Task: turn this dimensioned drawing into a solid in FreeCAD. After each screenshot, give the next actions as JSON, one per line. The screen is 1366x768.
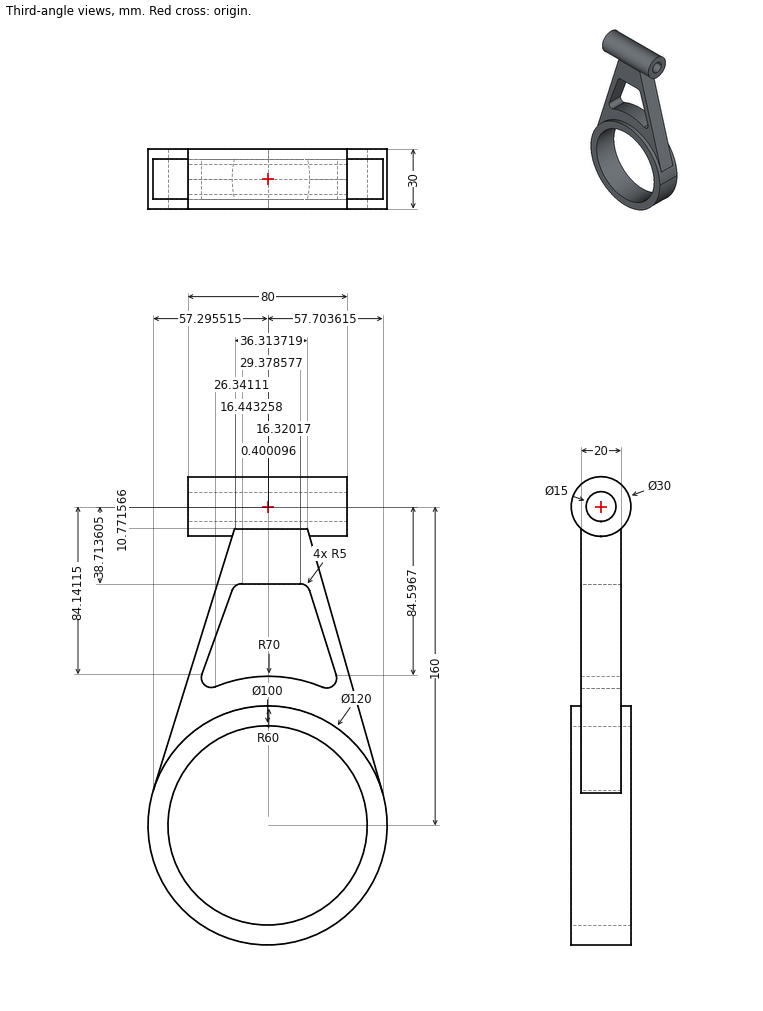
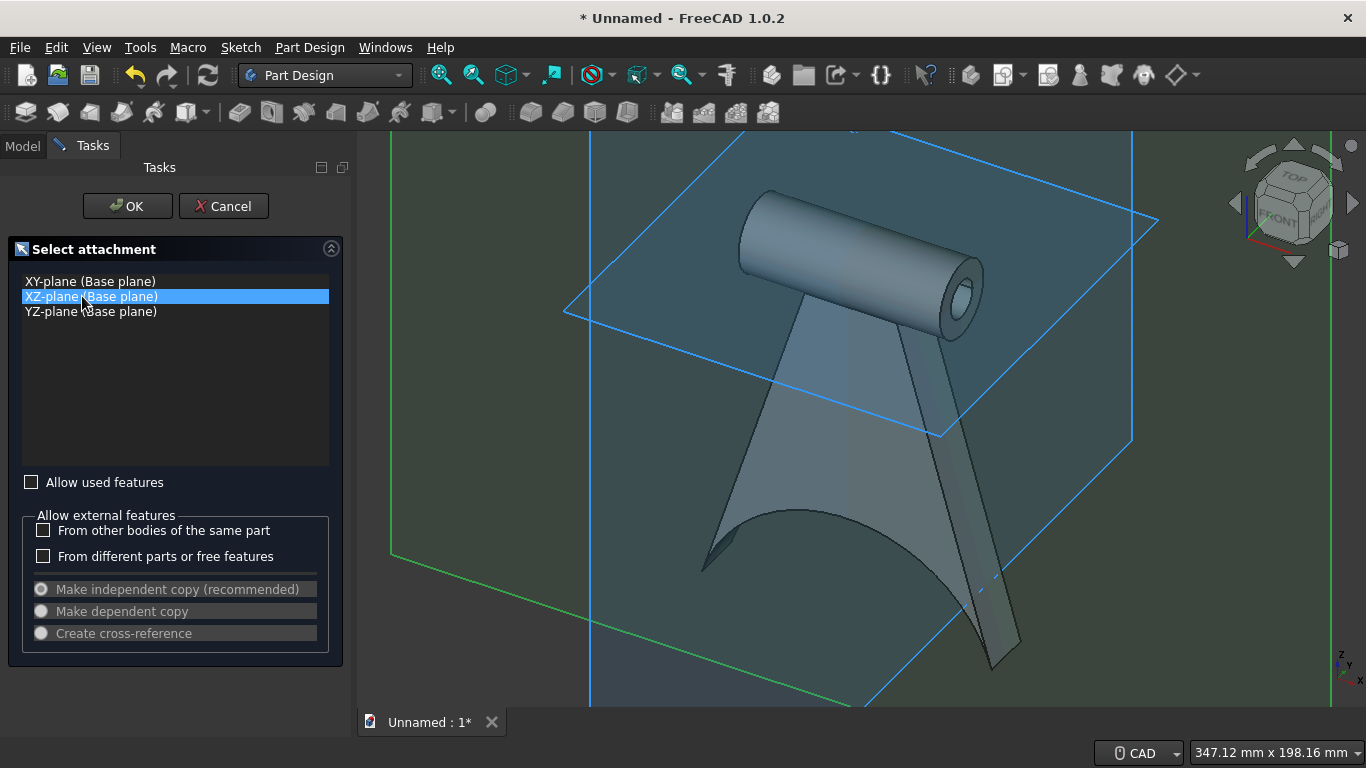
{"action": "left_click", "coordinate": [128, 206]}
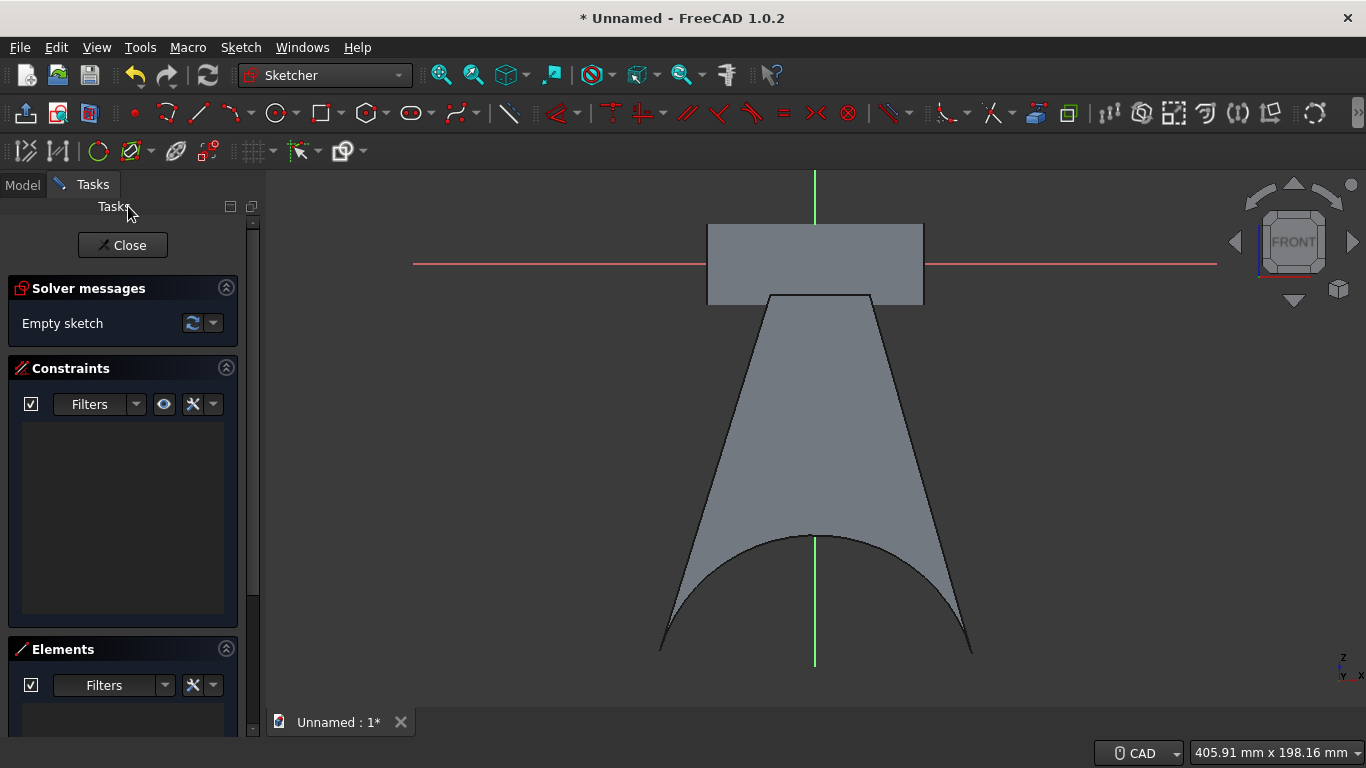
{"action": "key", "text": "q s"}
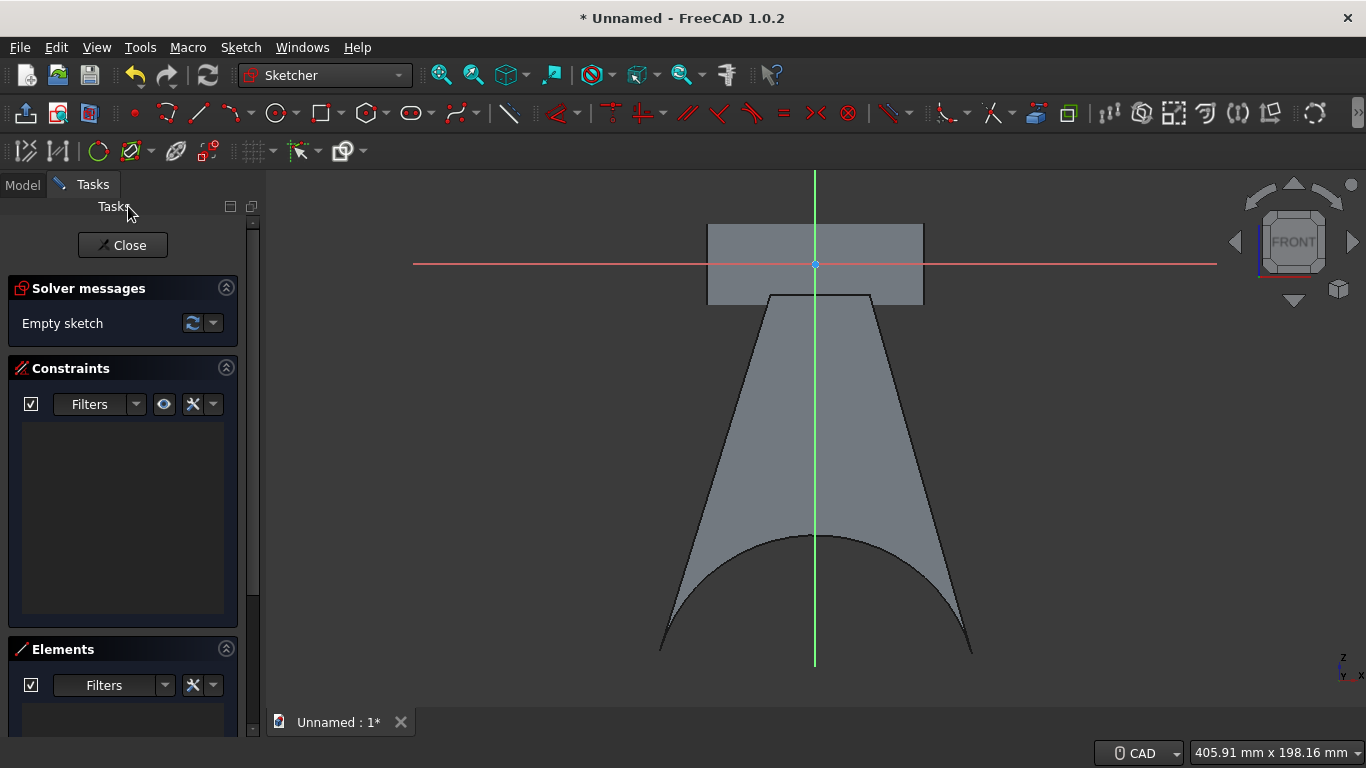
{"action": "scroll", "coordinate": [665, 288], "scroll_direction": "down", "scroll_amount": 3}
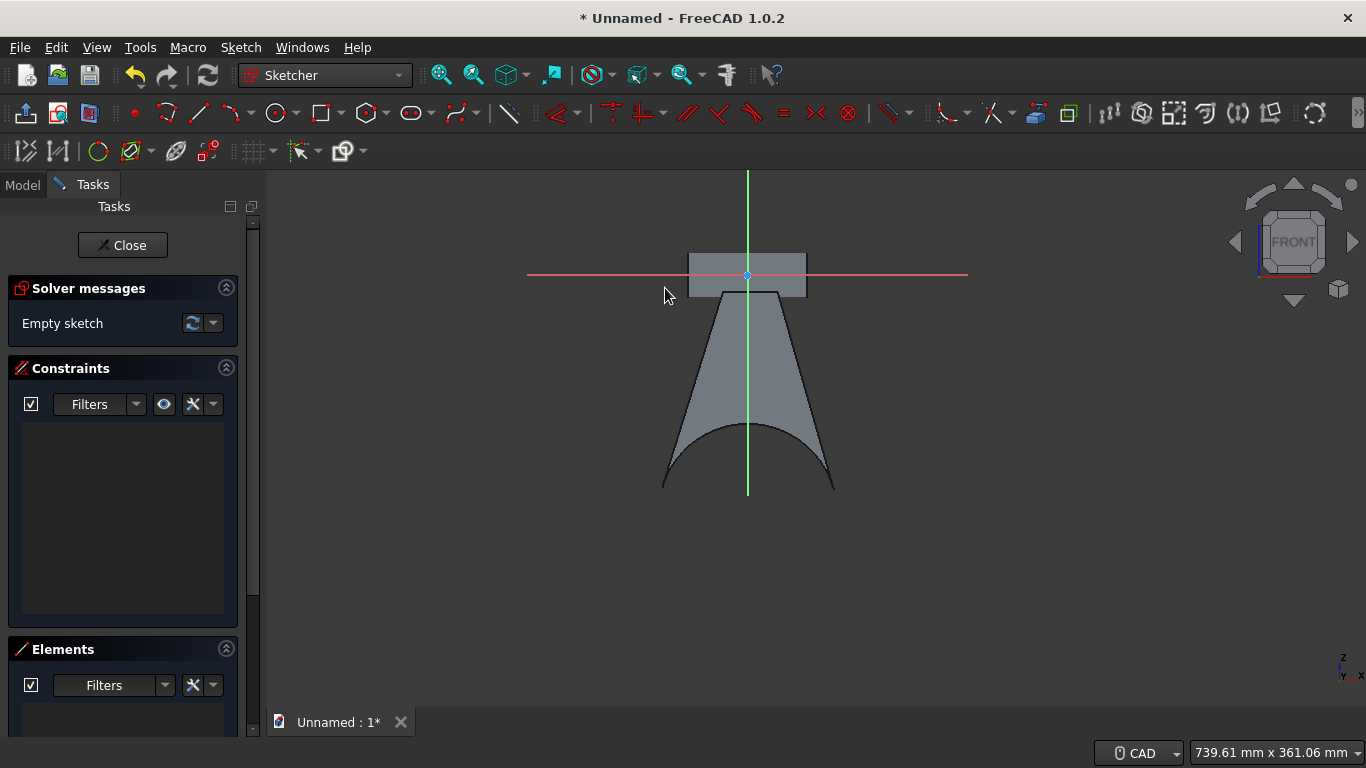
{"action": "left_click", "coordinate": [276, 114]}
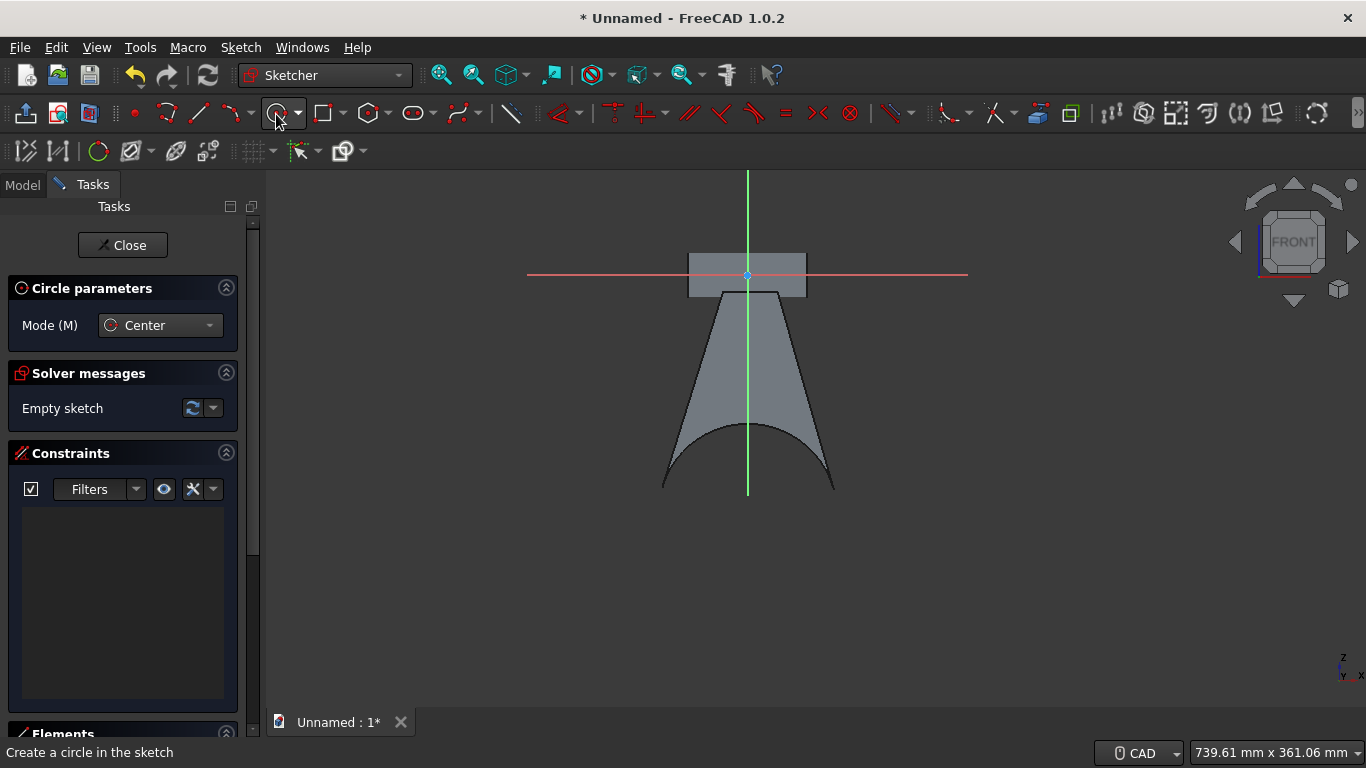
{"action": "left_click", "coordinate": [748, 513]}
{"action": "left_click", "coordinate": [811, 450]}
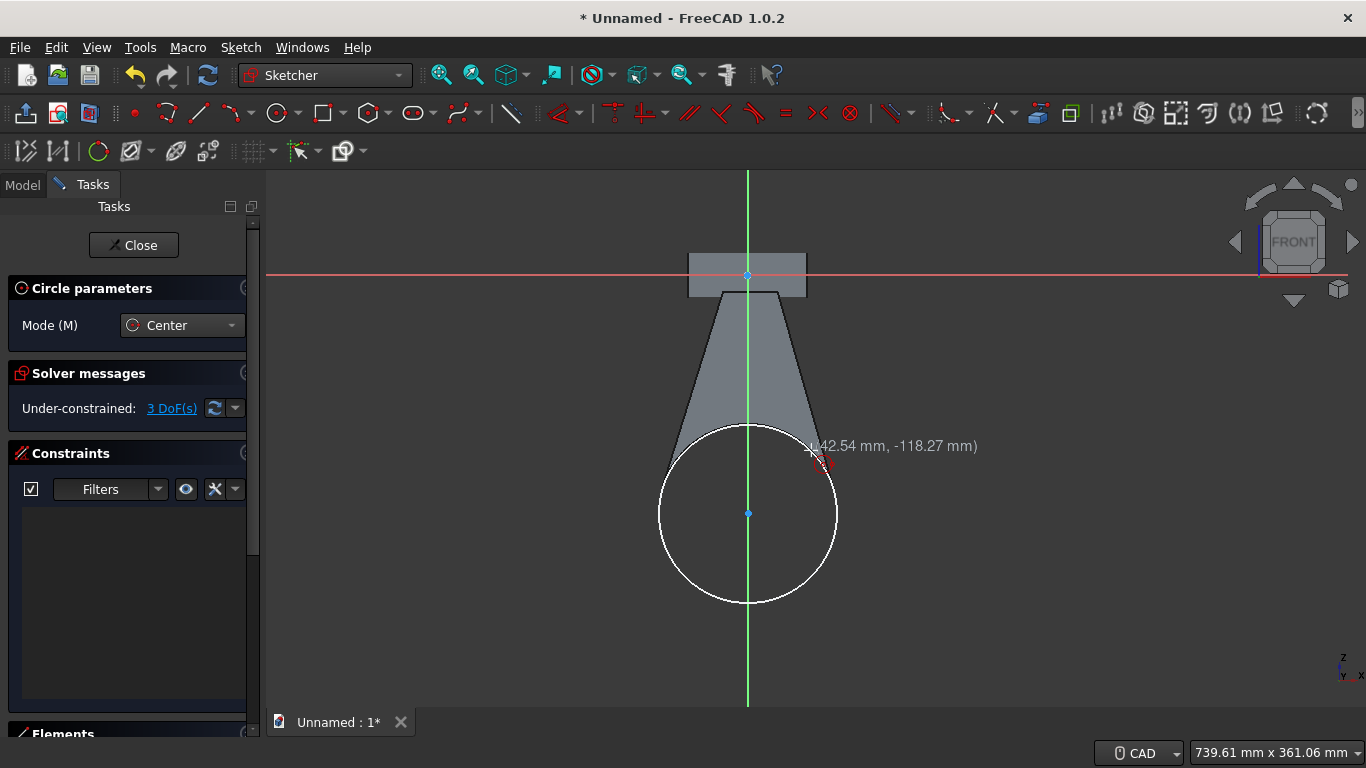
{"action": "left_click", "coordinate": [748, 514]}
{"action": "left_click", "coordinate": [800, 460]}
{"action": "key", "text": "Escape"}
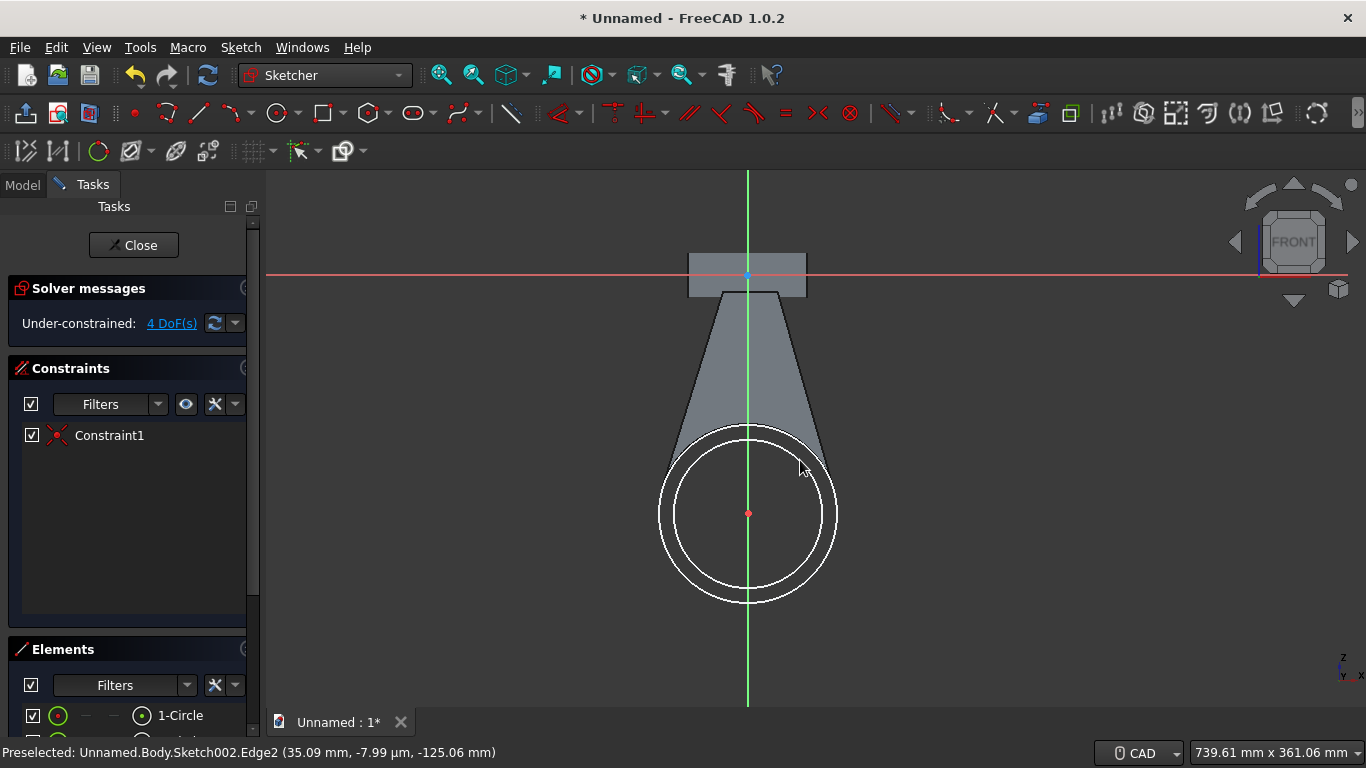
{"action": "left_click", "coordinate": [748, 514]}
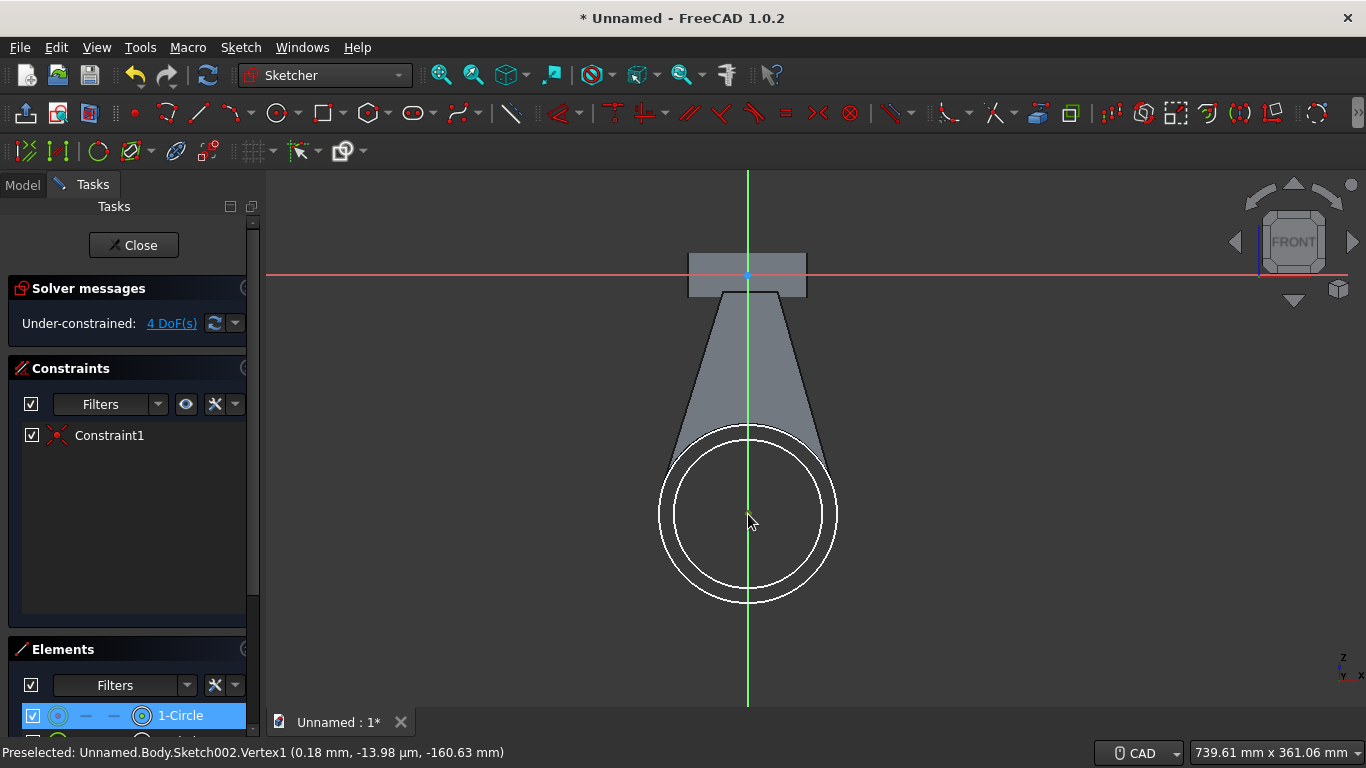
{"action": "left_click", "coordinate": [748, 645]}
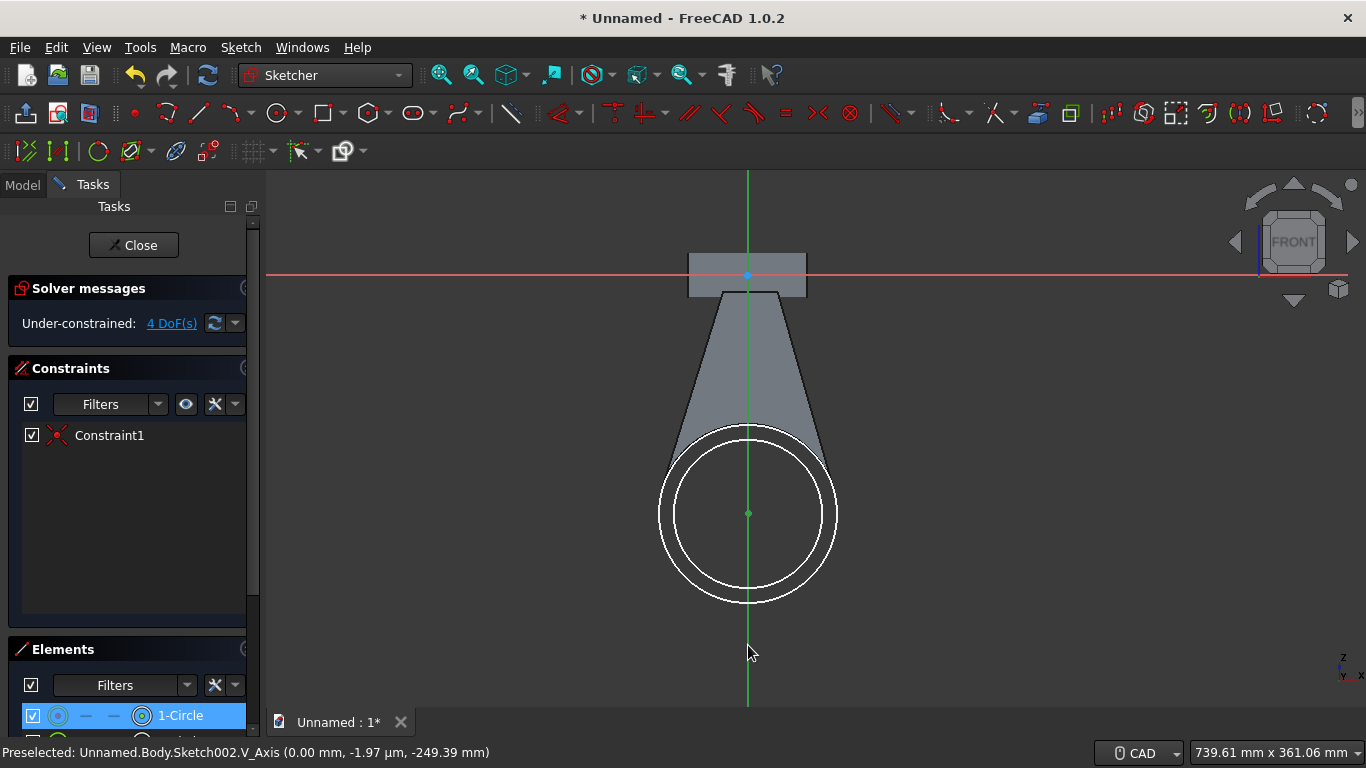
{"action": "left_click", "coordinate": [614, 114]}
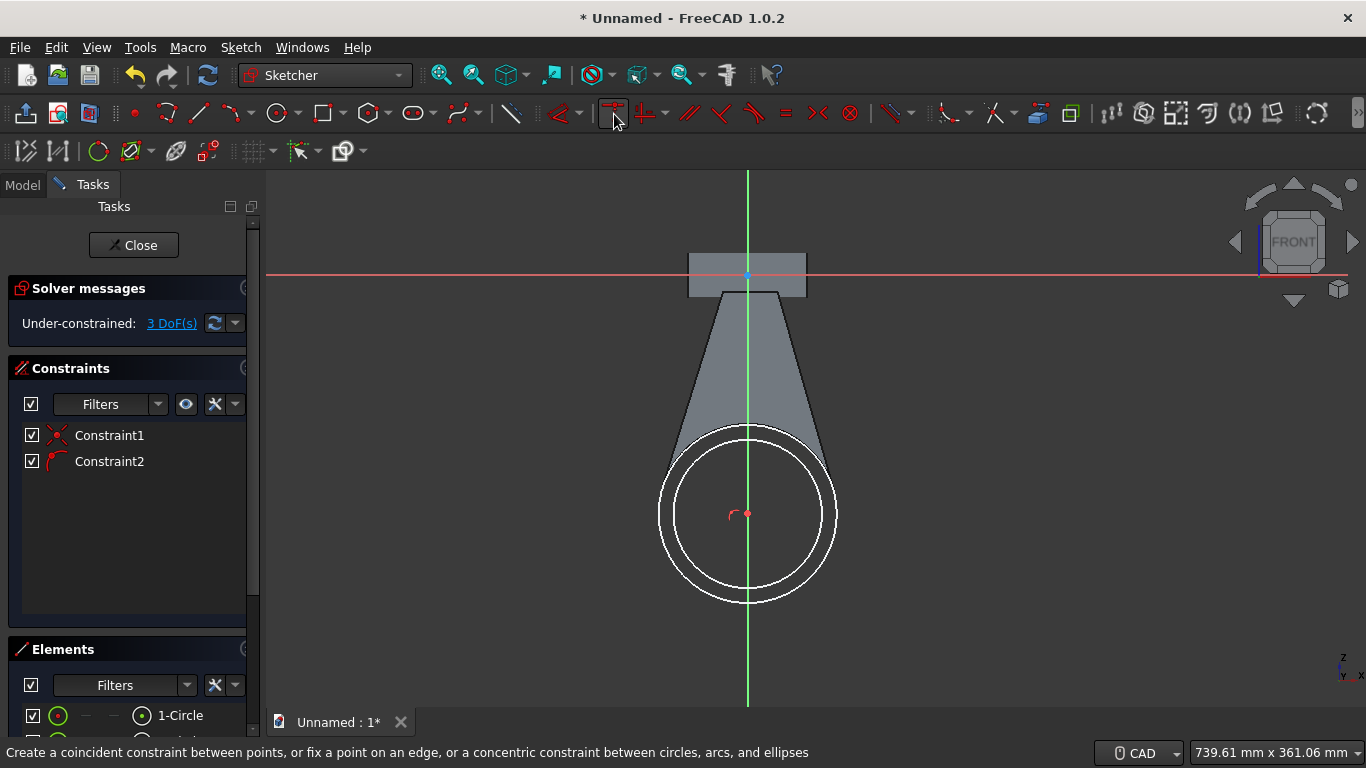
{"action": "key", "text": "d"}